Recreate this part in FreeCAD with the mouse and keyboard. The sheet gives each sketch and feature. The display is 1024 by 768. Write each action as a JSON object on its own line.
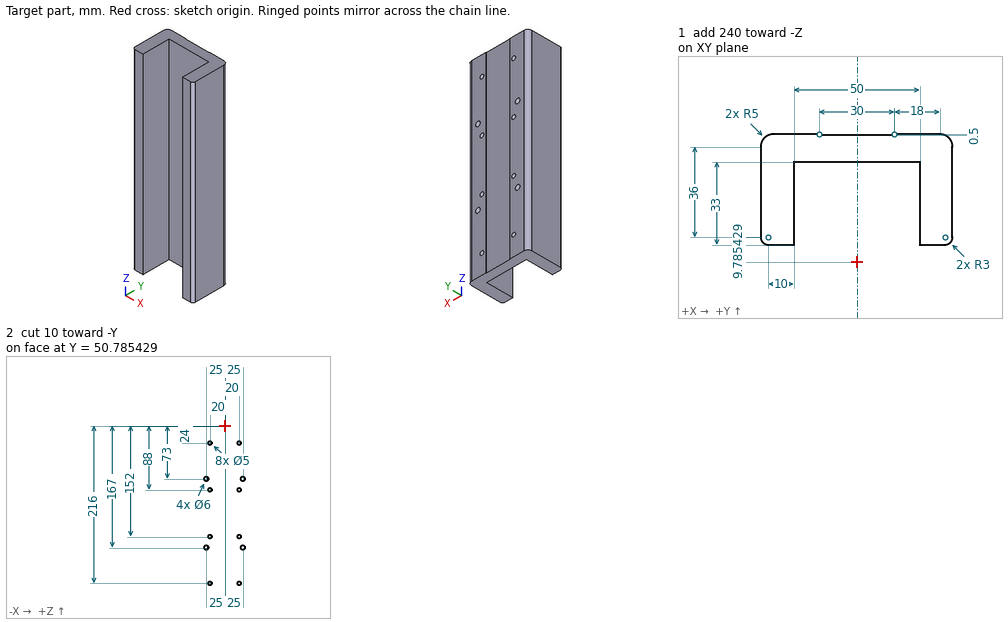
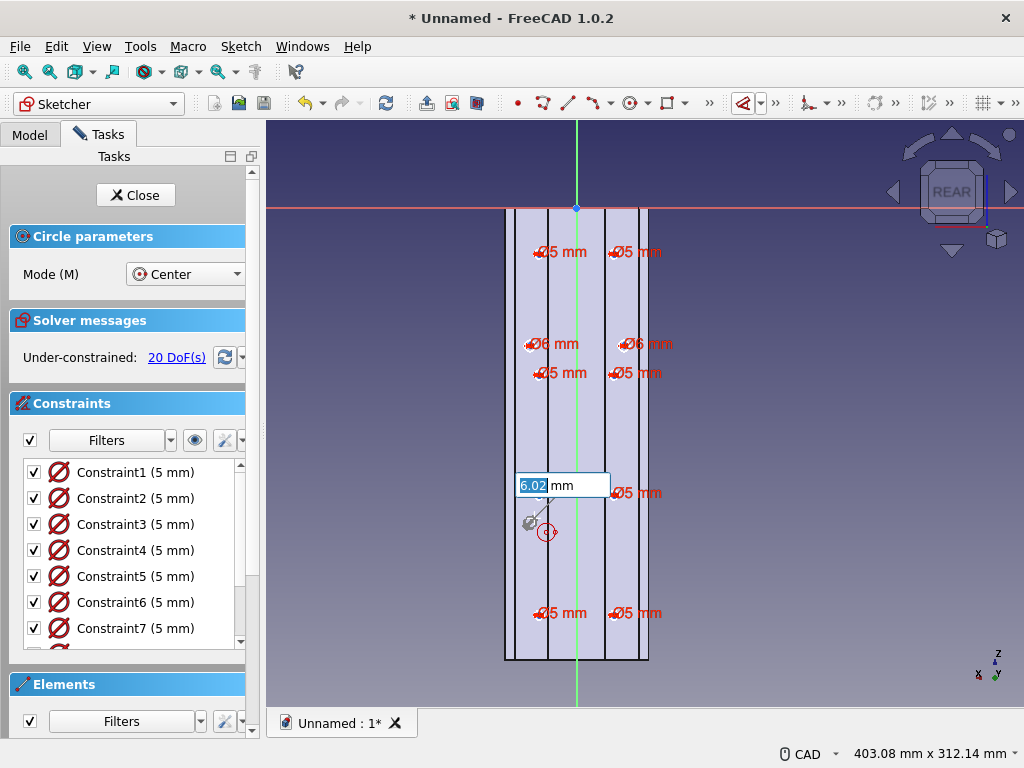
{"action": "type", "text": "6"}
{"action": "key", "text": "Return"}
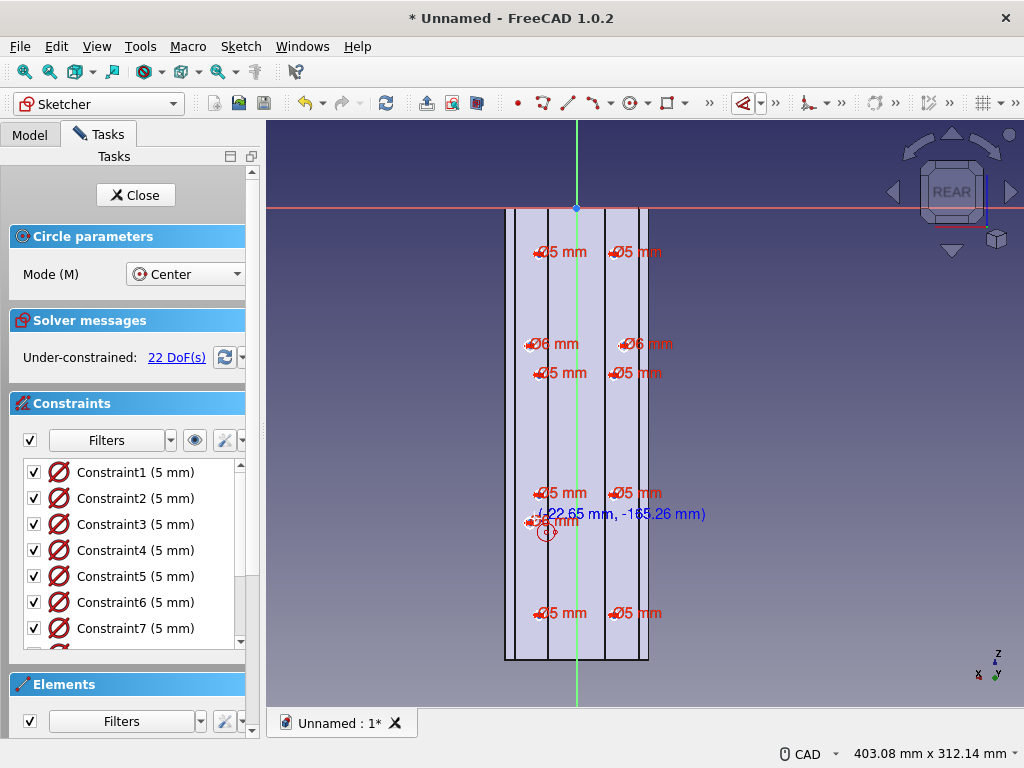
{"action": "scroll", "coordinate": [624, 522], "scroll_direction": "up", "scroll_amount": 7}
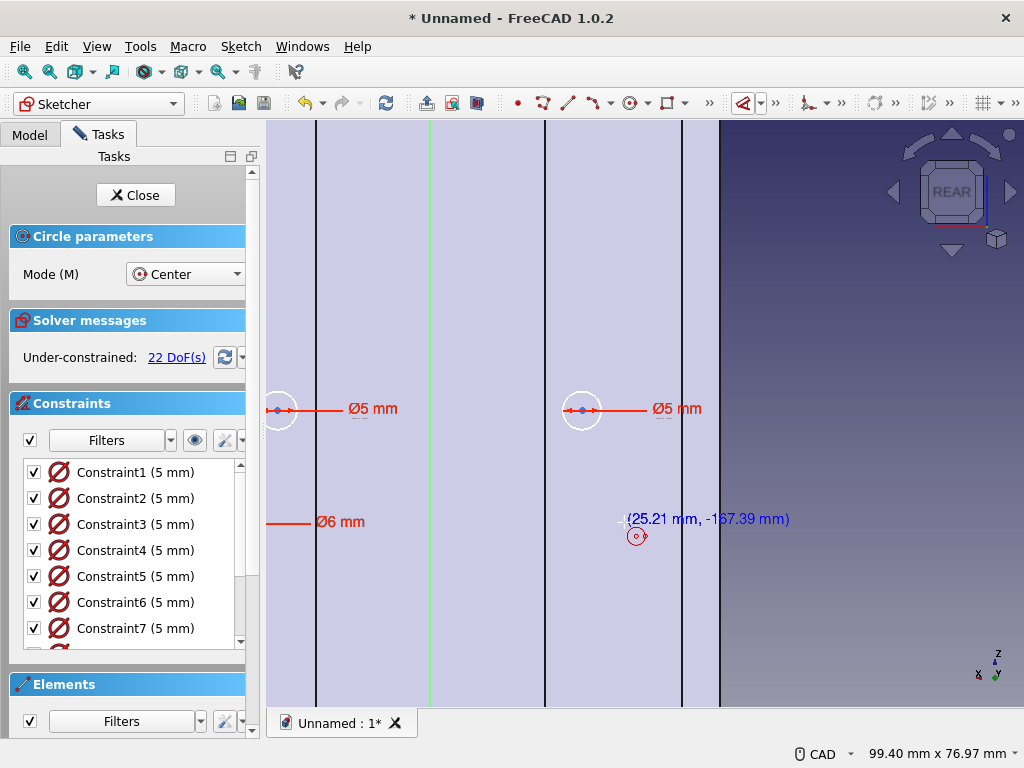
{"action": "scroll", "coordinate": [624, 522], "scroll_direction": "down", "scroll_amount": 7}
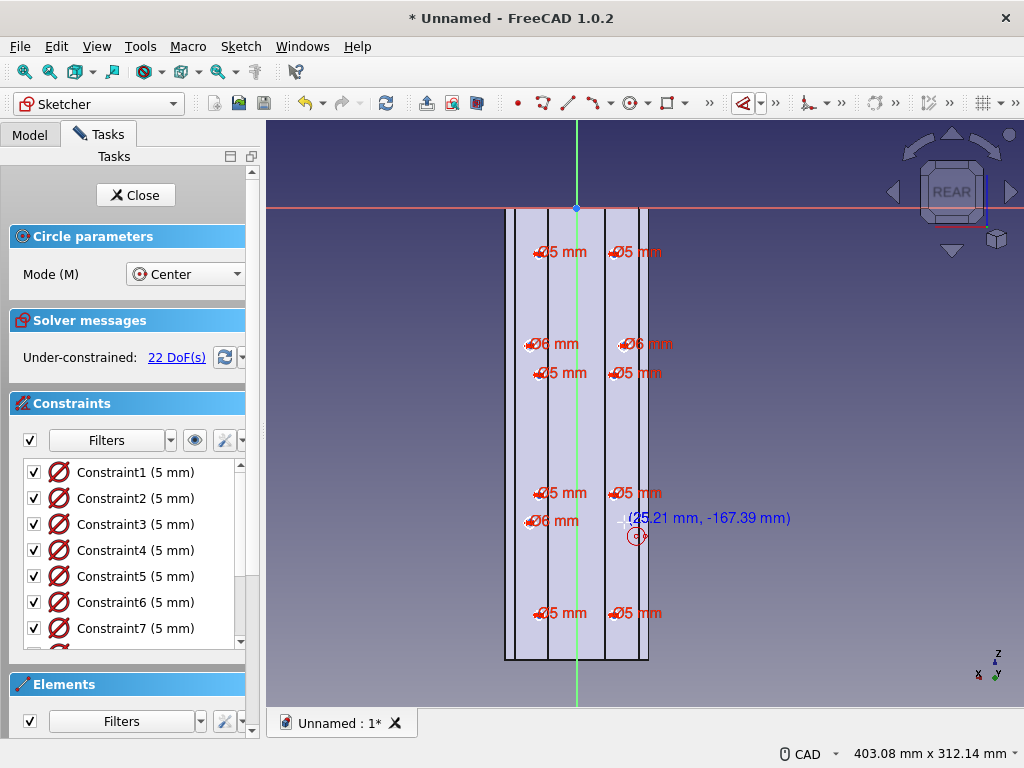
{"action": "left_click", "coordinate": [624, 522]}
{"action": "mouse_move", "coordinate": [628, 518]}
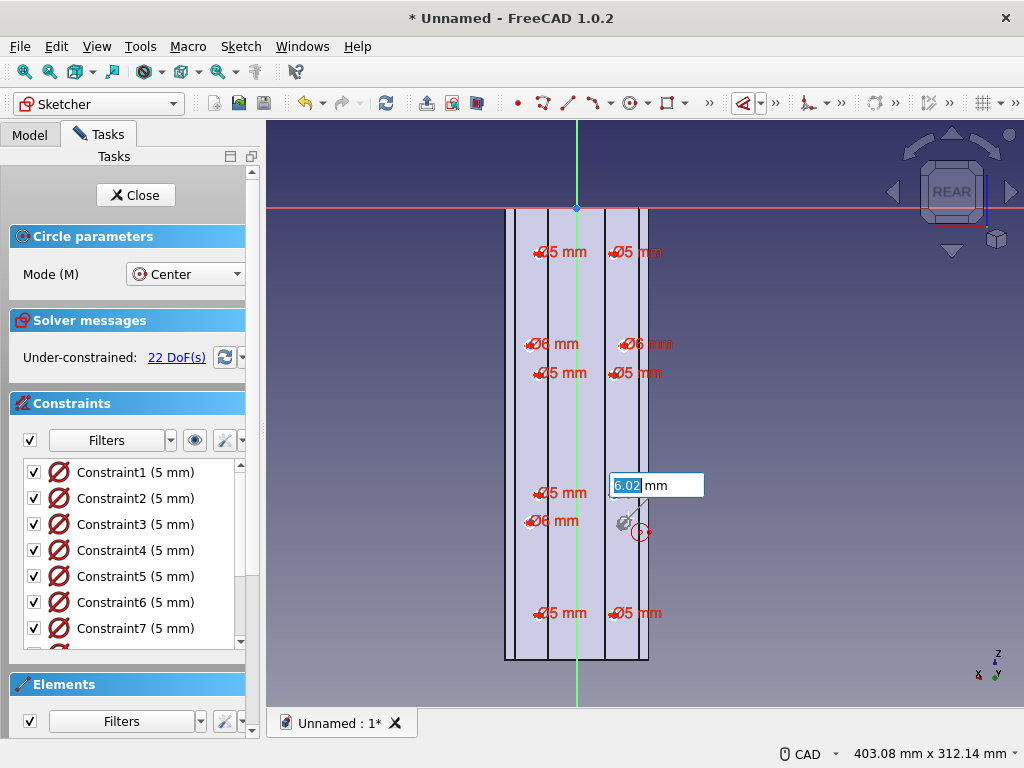
{"action": "type", "text": "6"}
{"action": "key", "text": "Return"}
{"action": "key", "text": "Escape"}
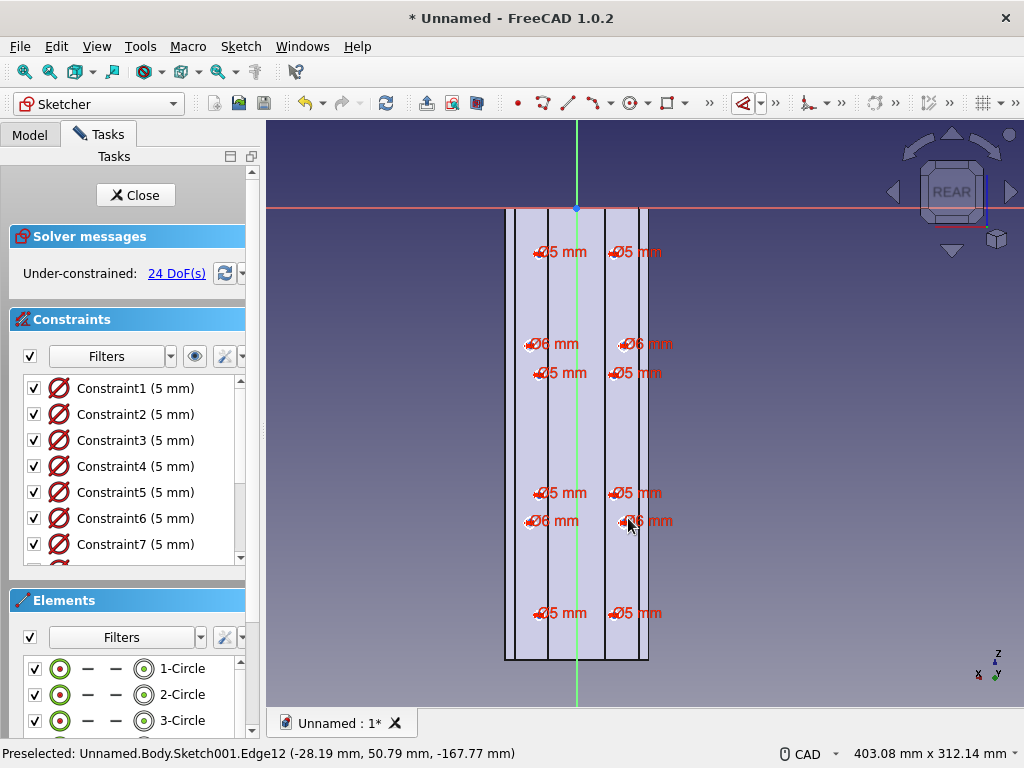
{"action": "left_click", "coordinate": [539, 254]}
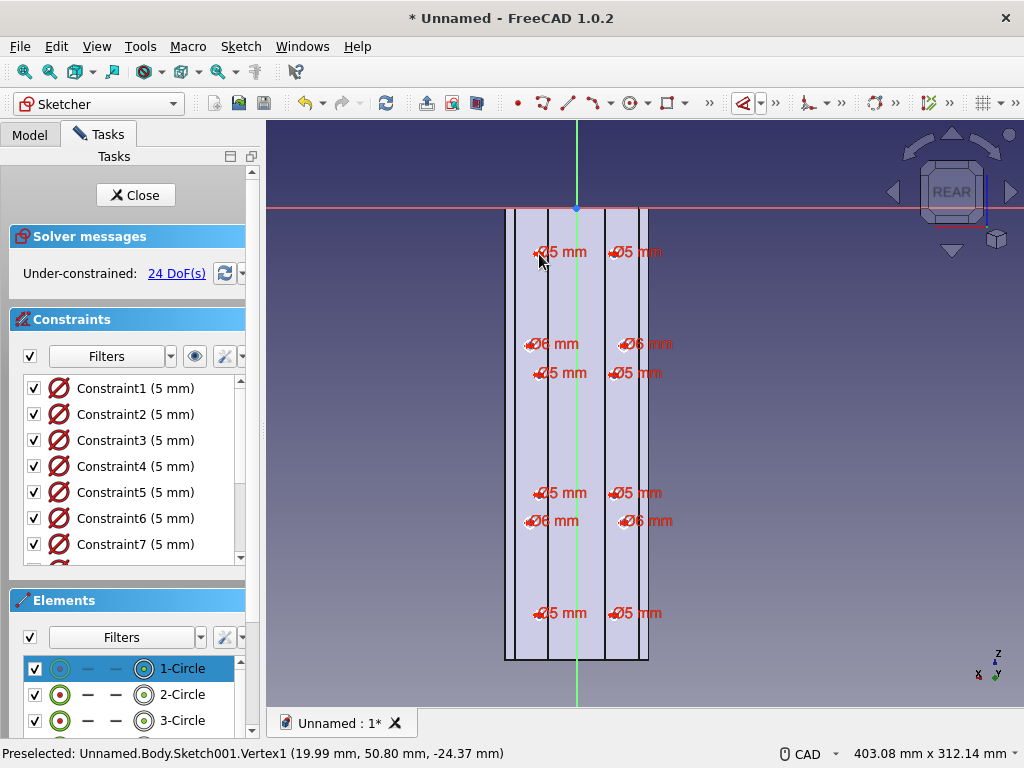
{"action": "left_click", "coordinate": [614, 254]}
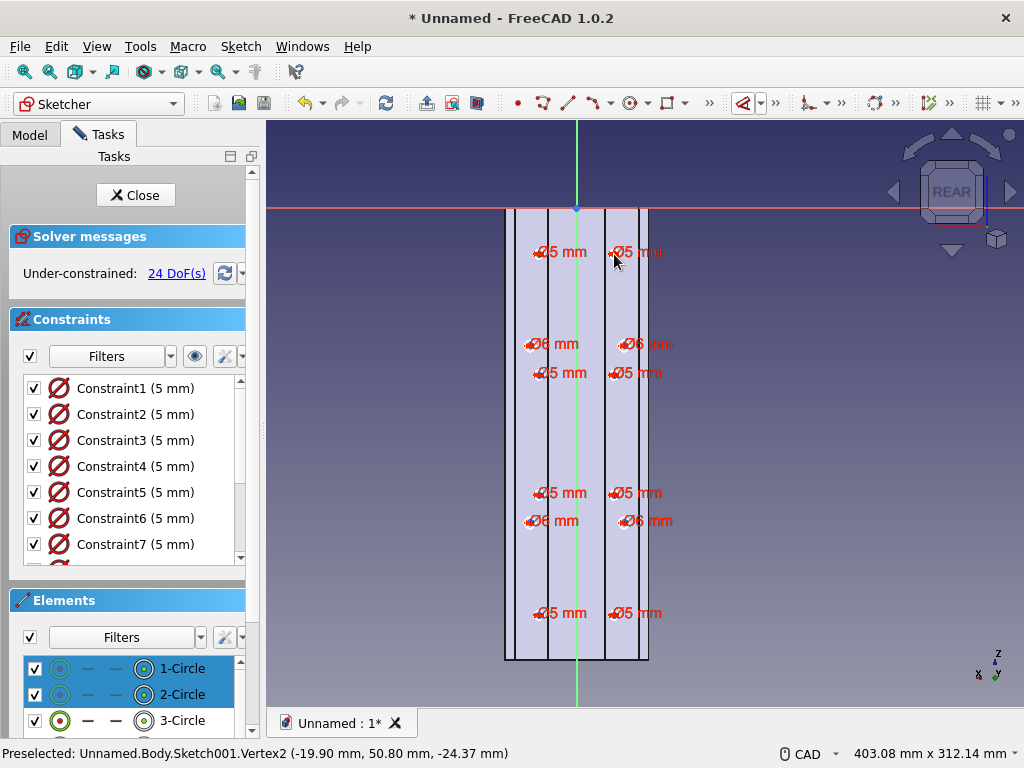
{"action": "key", "text": "h"}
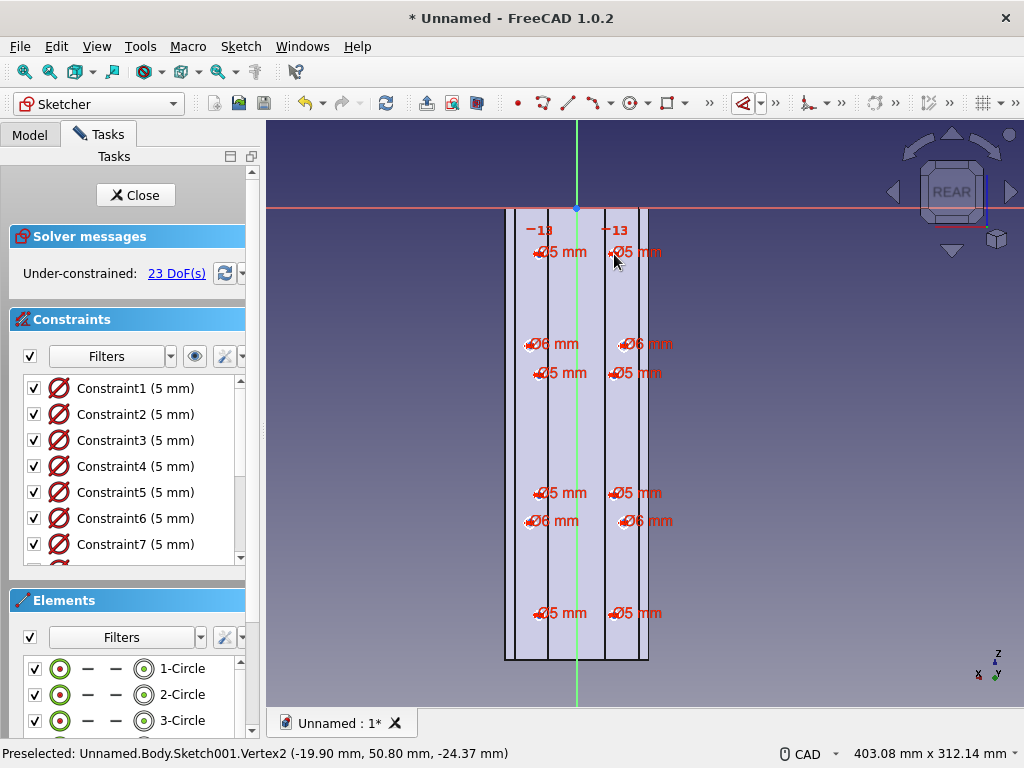
{"action": "left_click", "coordinate": [539, 254]}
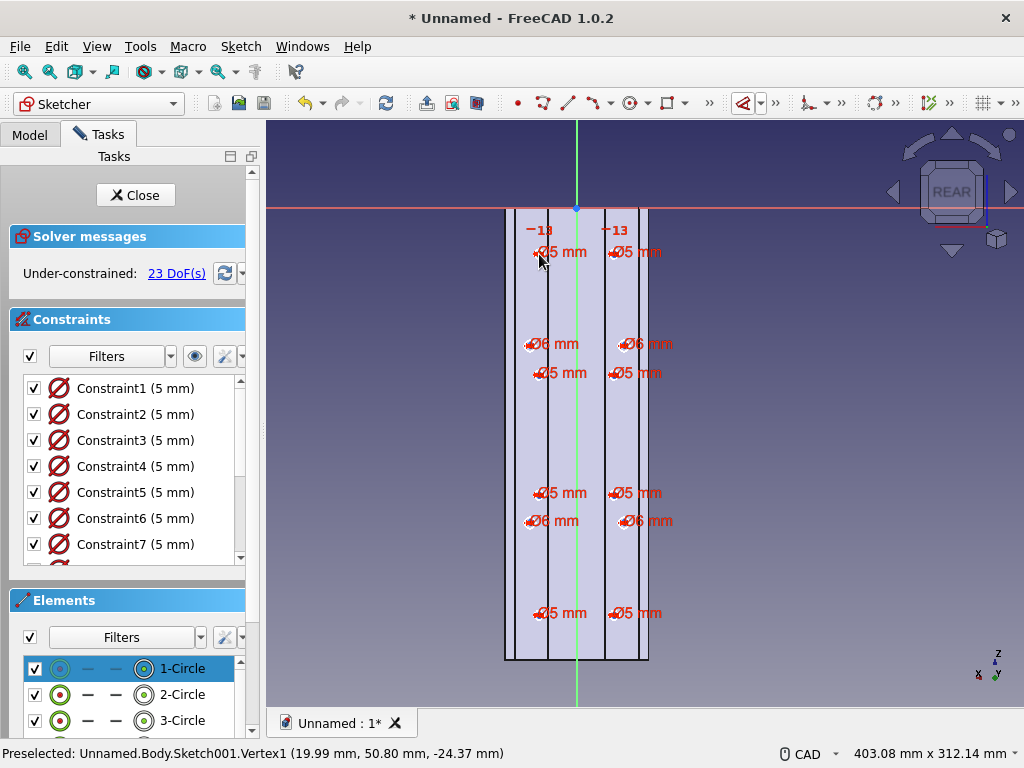
{"action": "left_click", "coordinate": [539, 375]}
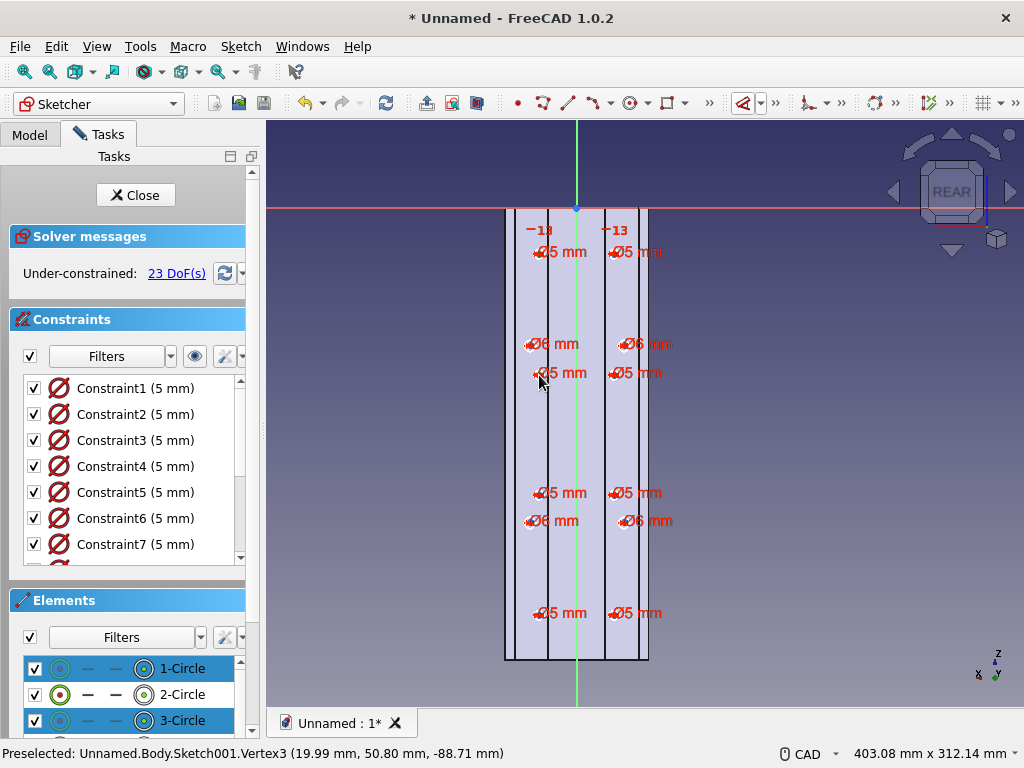
{"action": "key", "text": "v"}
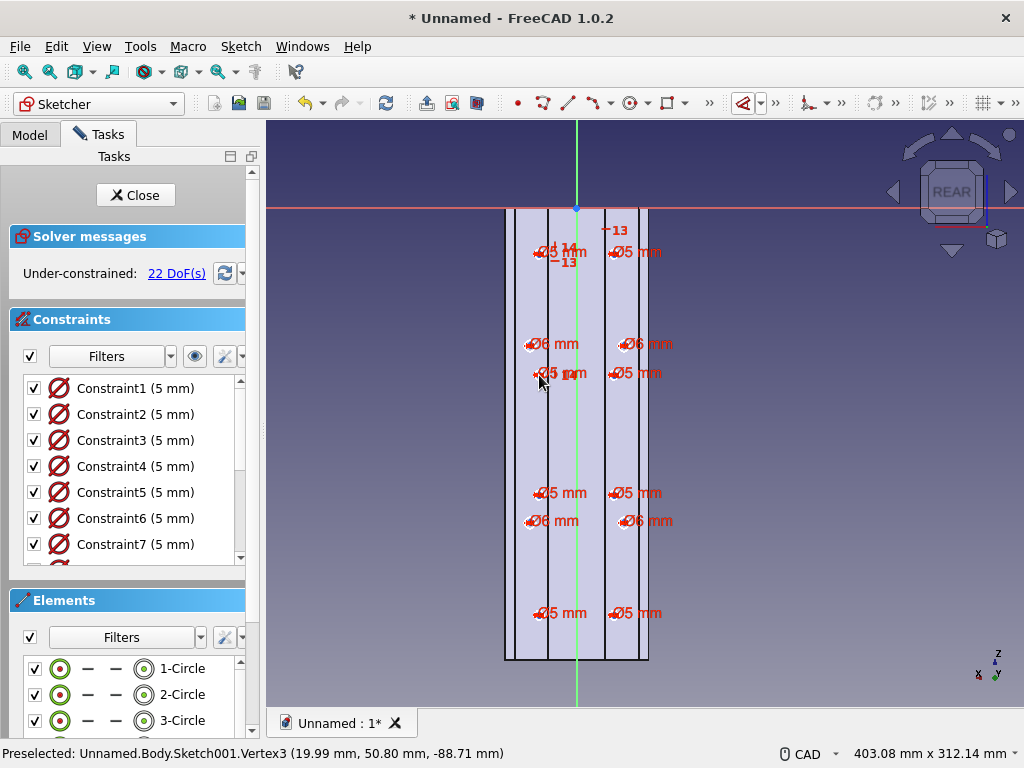
{"action": "left_click", "coordinate": [614, 254]}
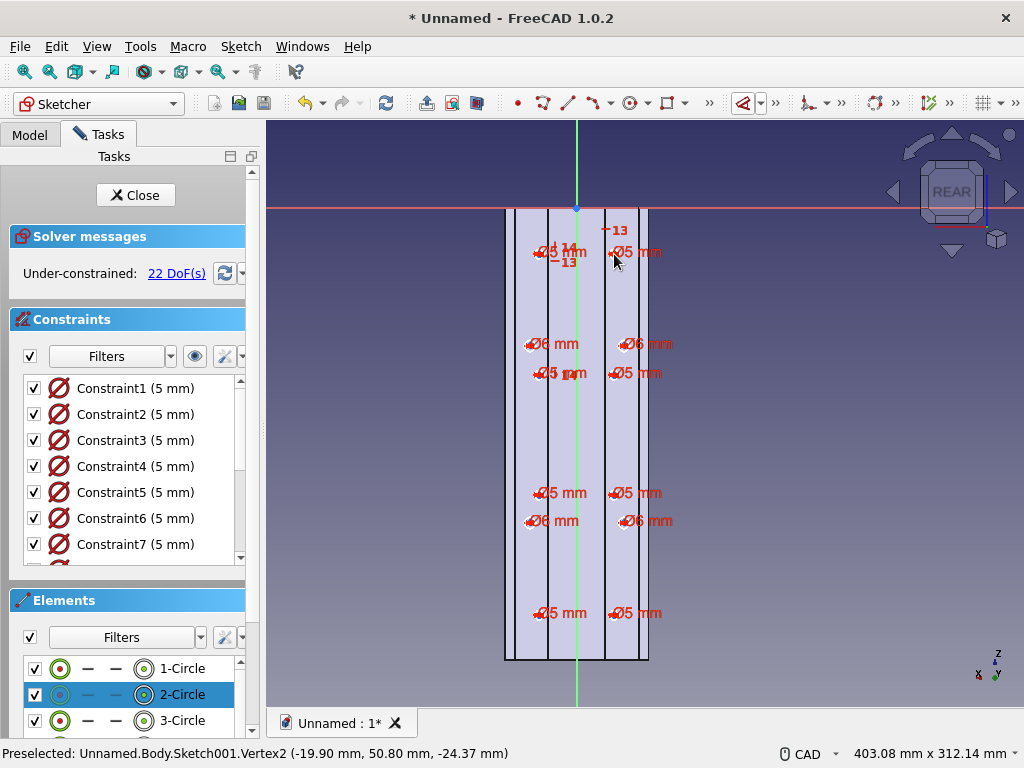
{"action": "left_click", "coordinate": [614, 375]}